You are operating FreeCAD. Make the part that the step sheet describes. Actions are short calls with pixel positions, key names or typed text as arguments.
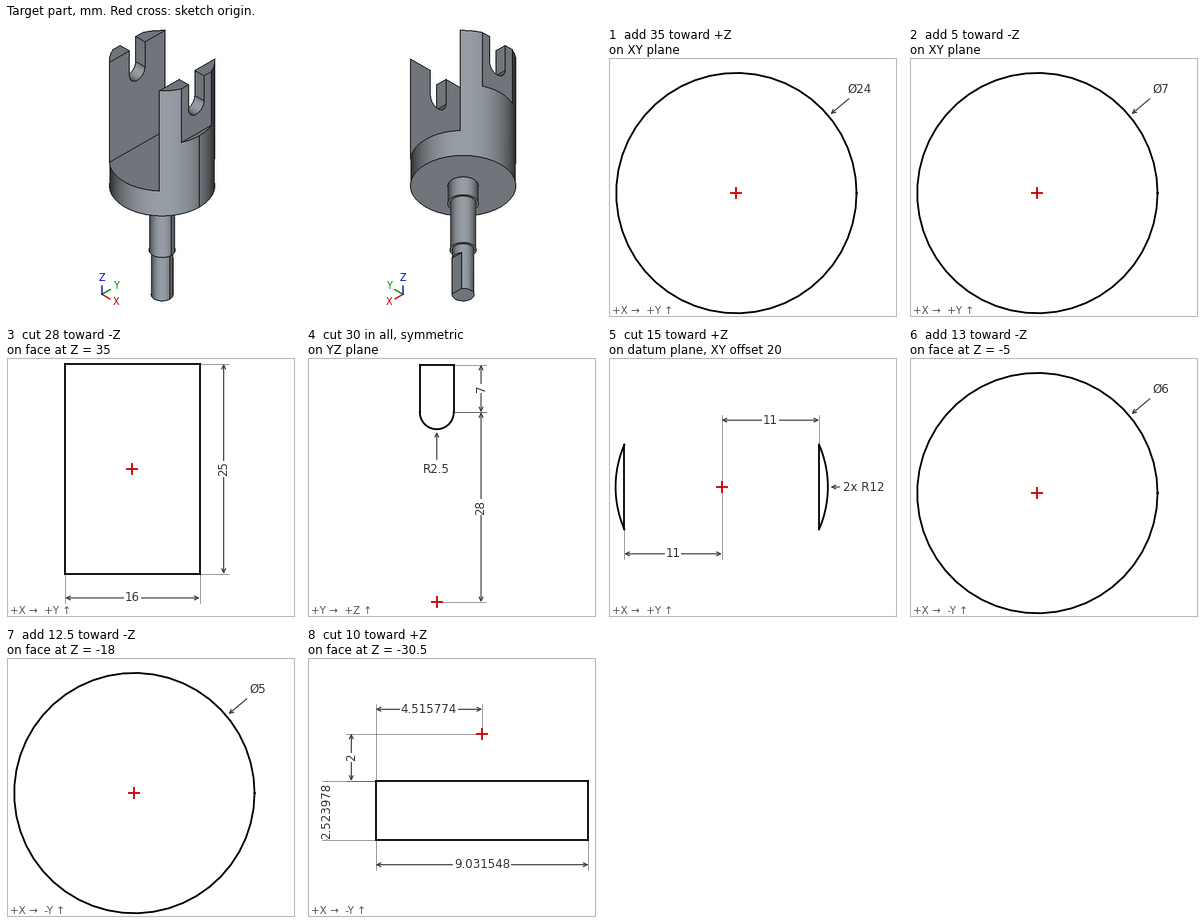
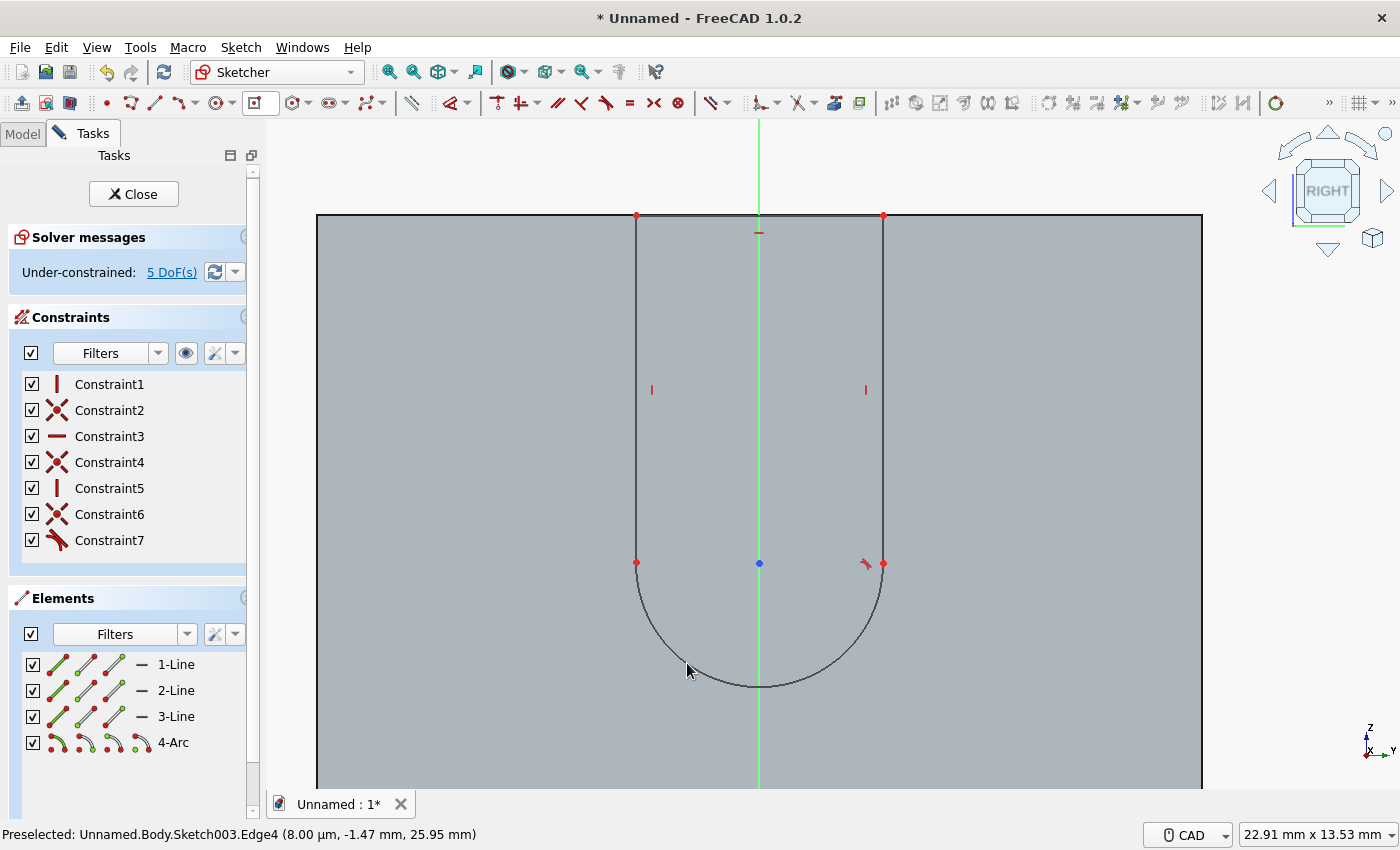
click(636, 320)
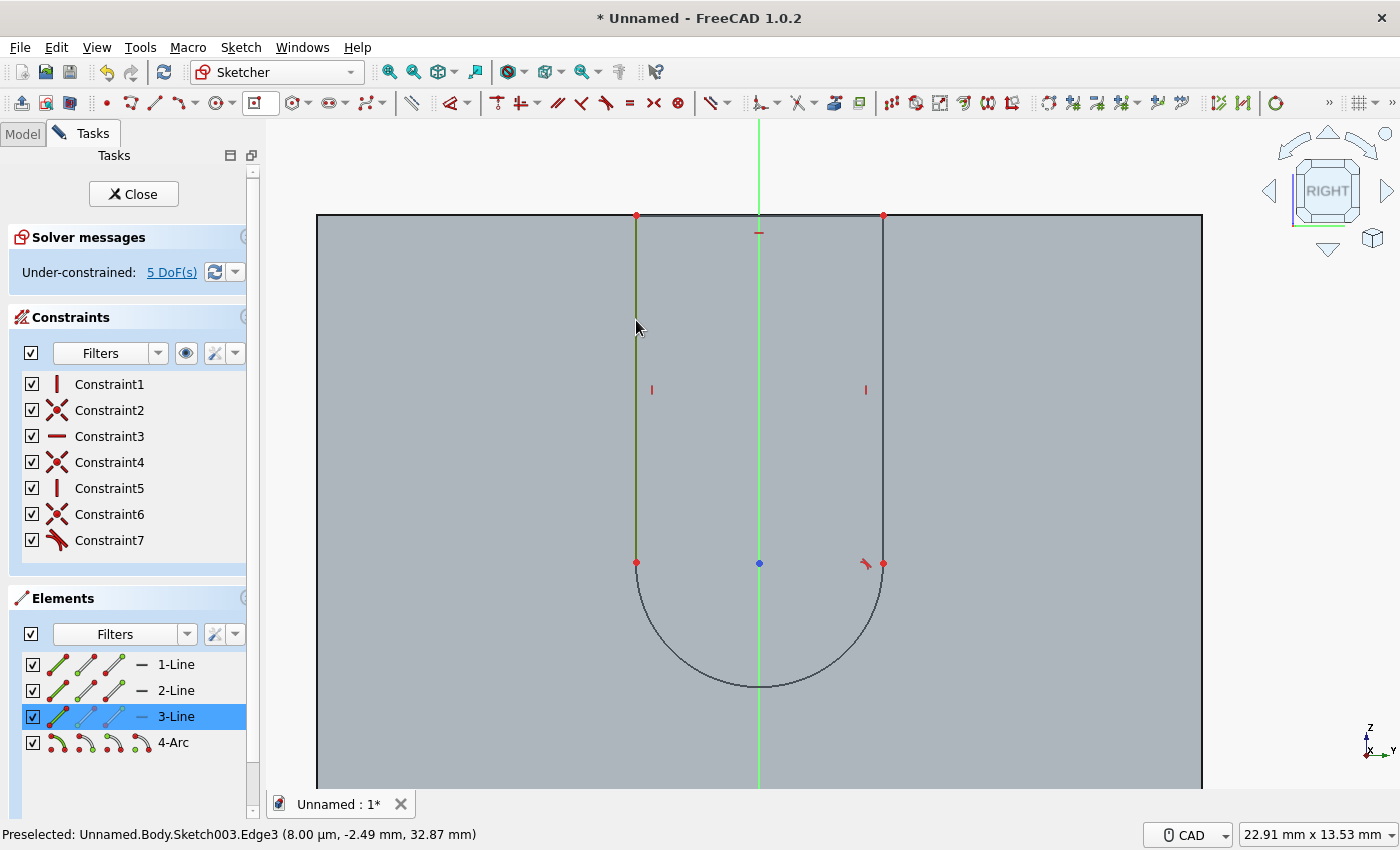
click(687, 663)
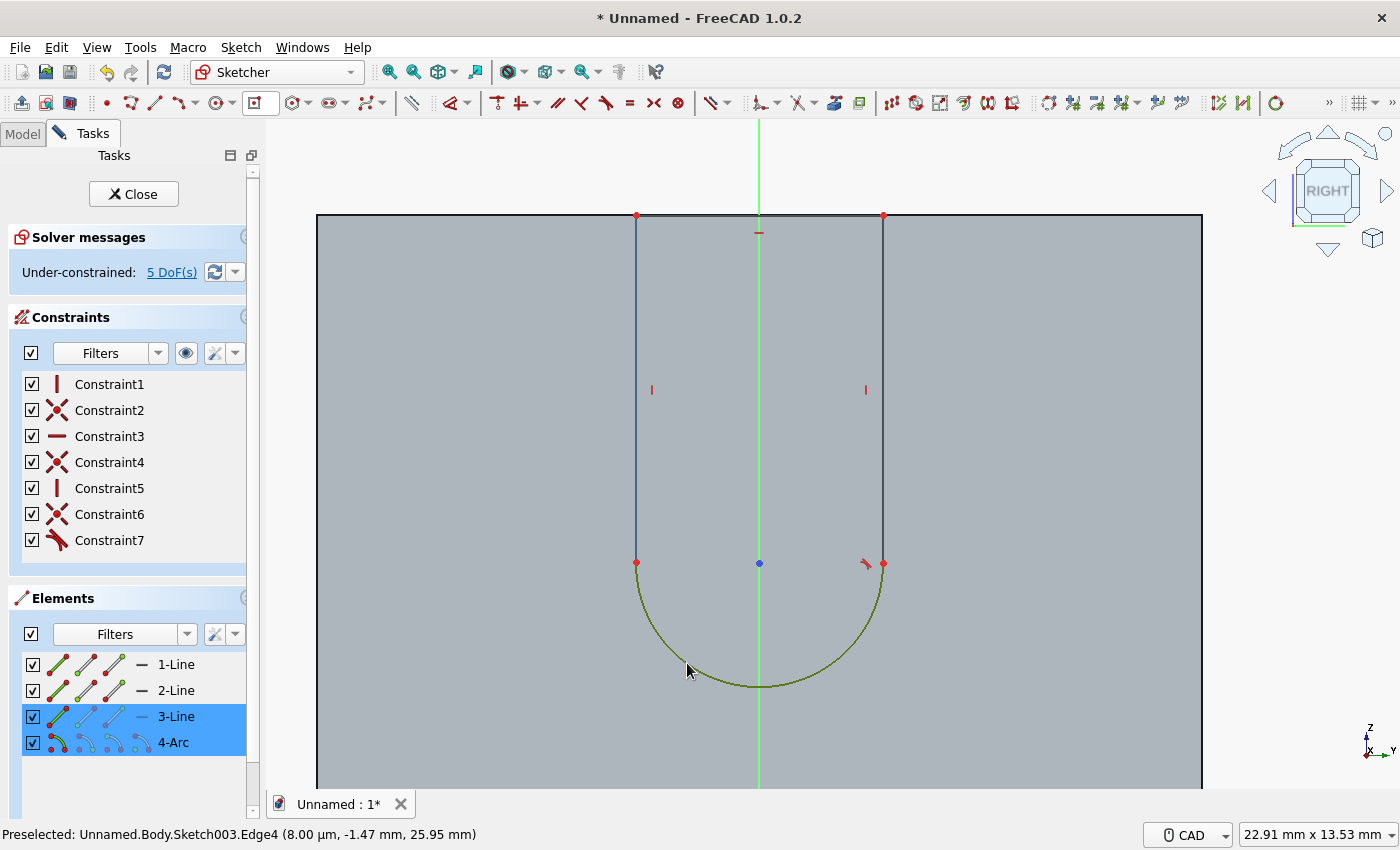
click(606, 104)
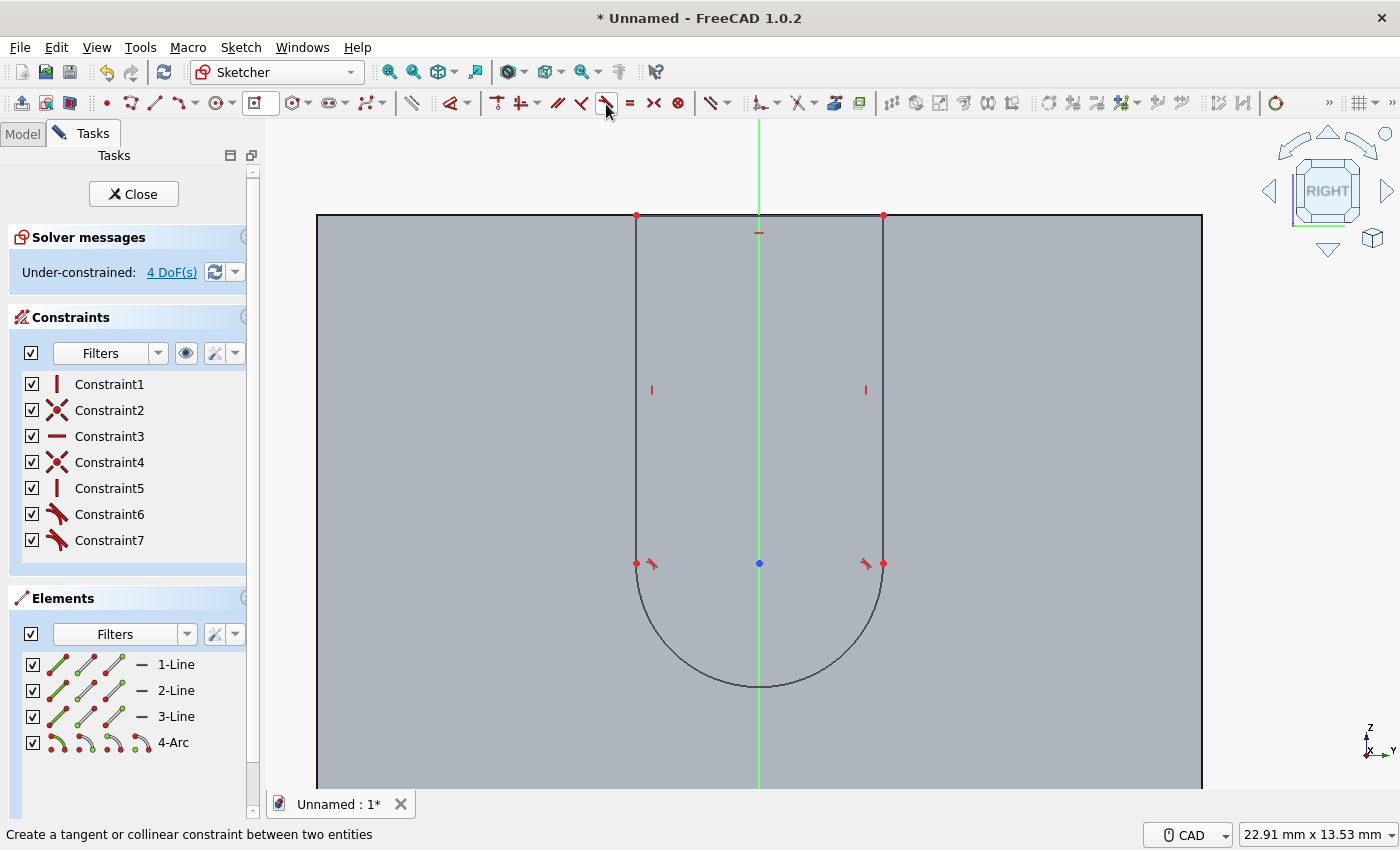
click(760, 564)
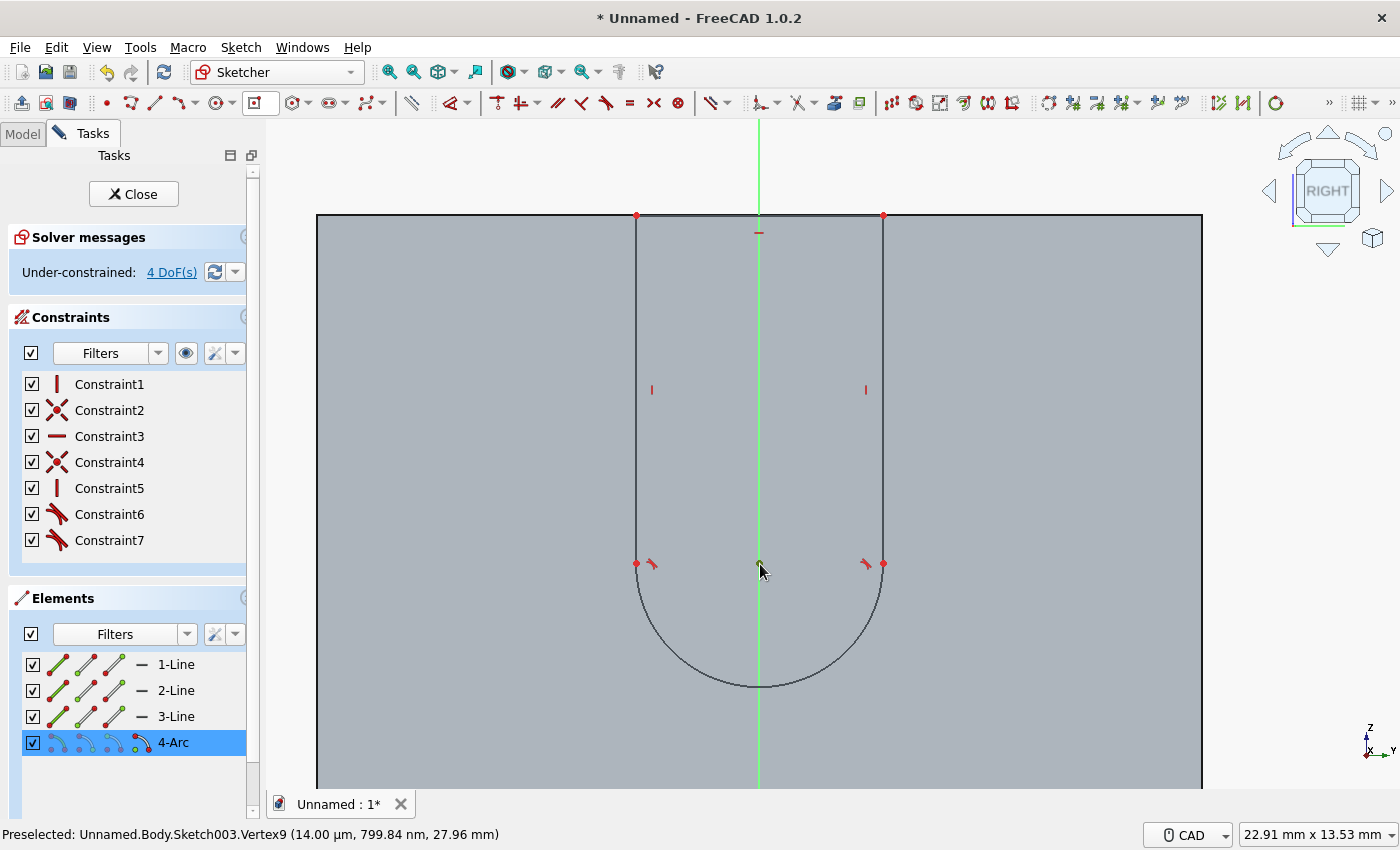
click(759, 629)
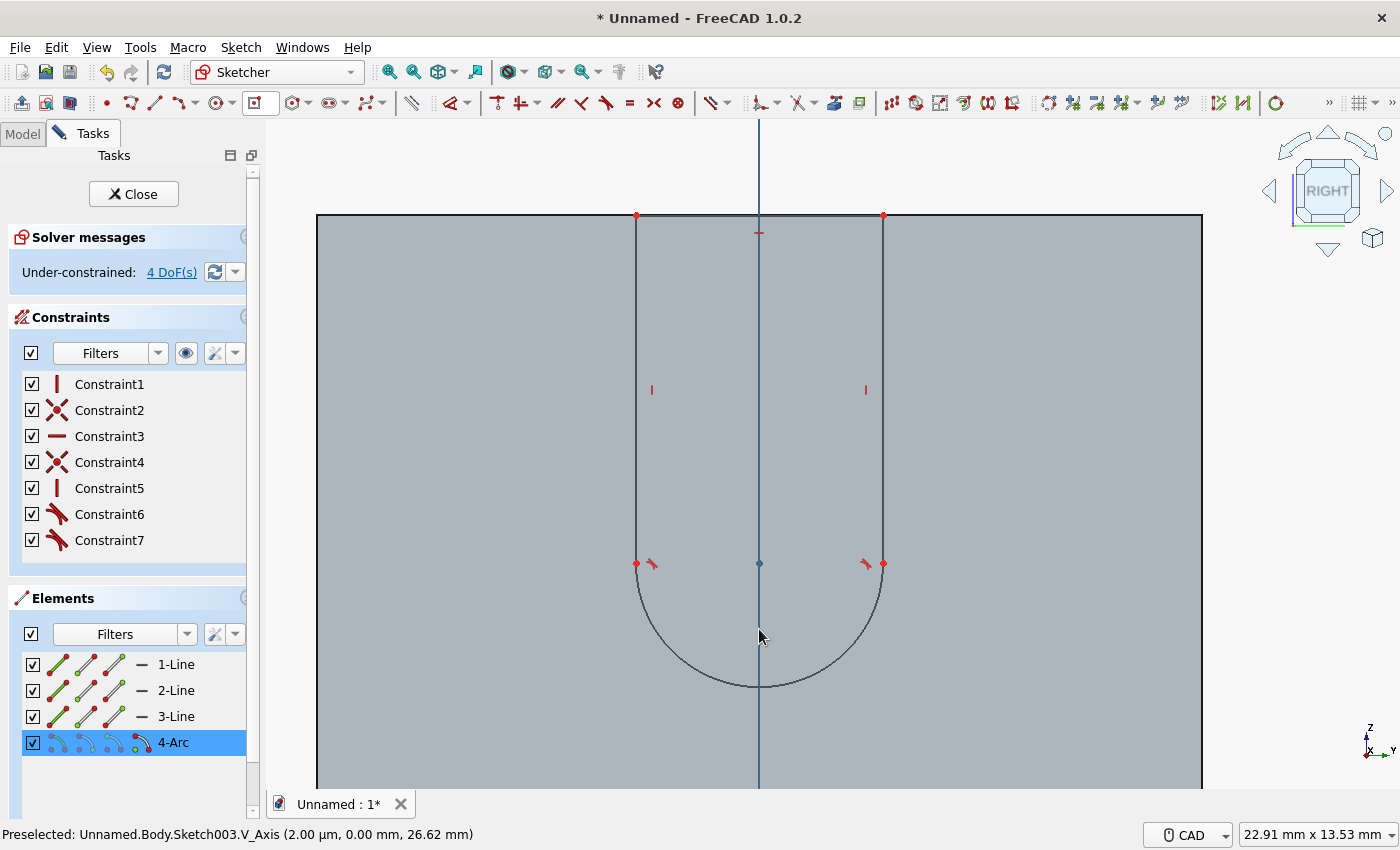
click(498, 104)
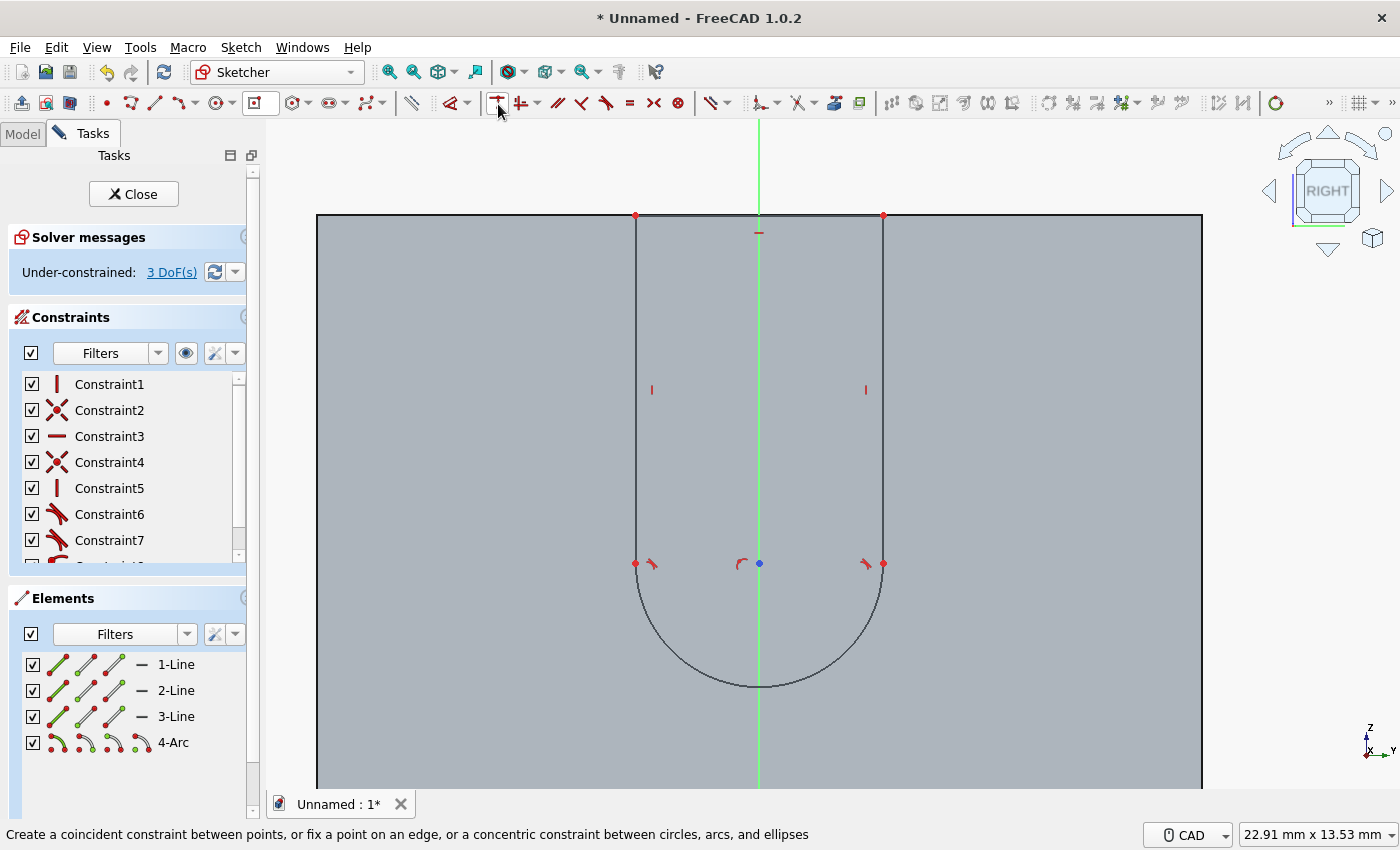
click(450, 104)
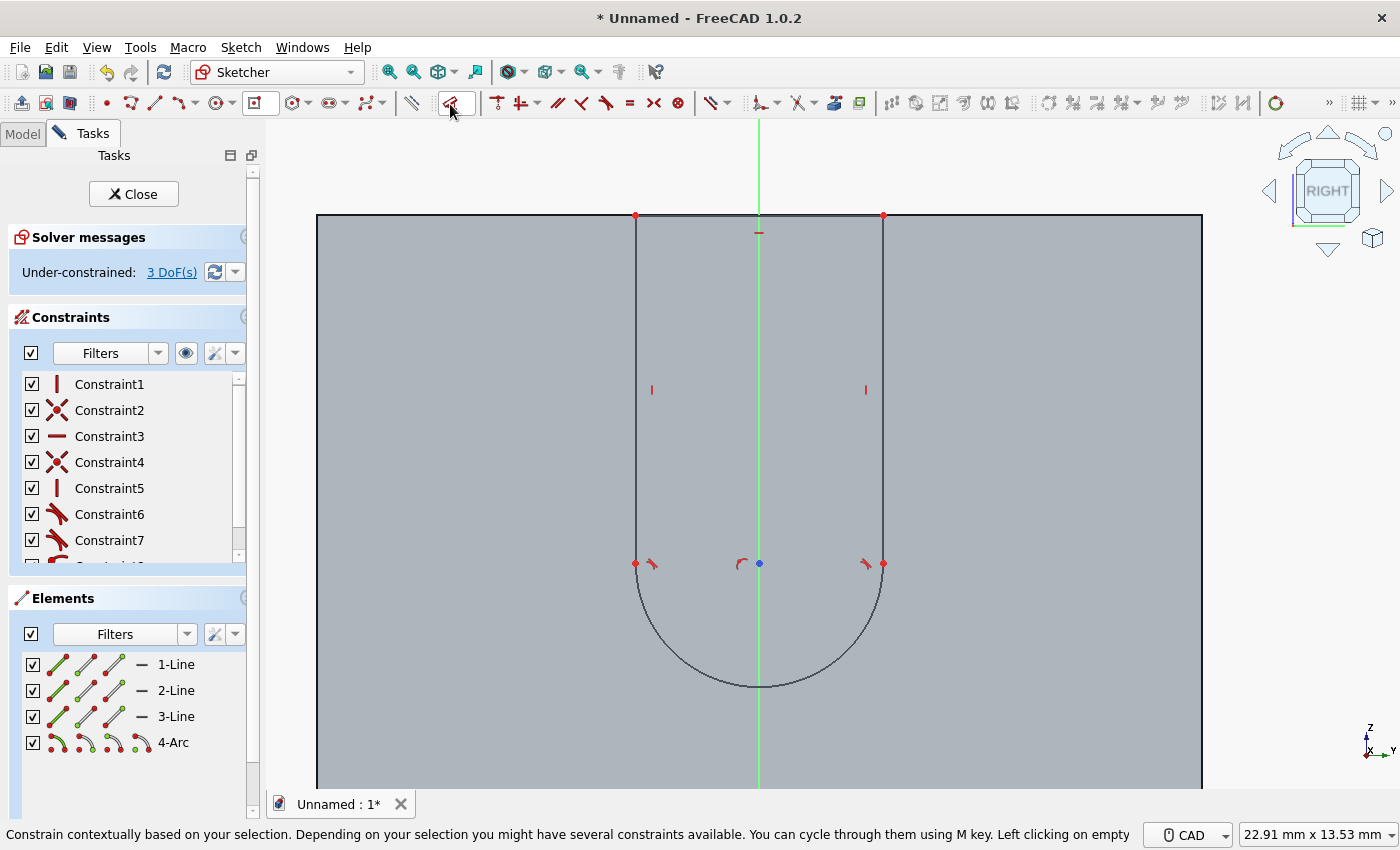
click(687, 664)
click(668, 690)